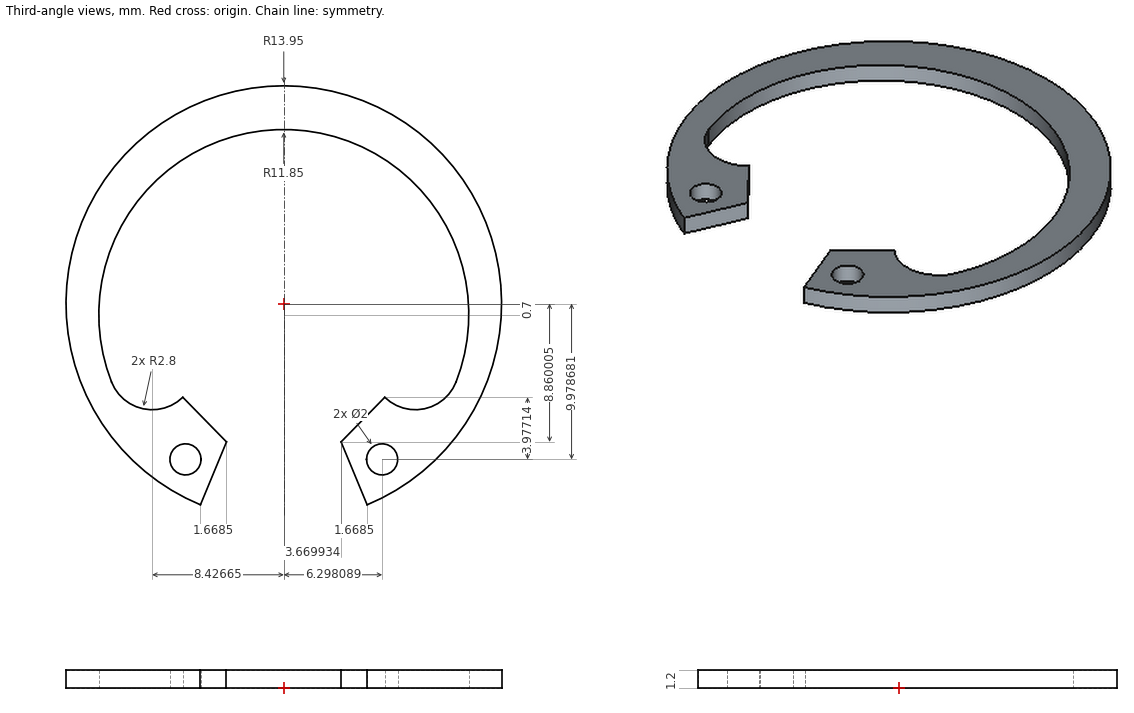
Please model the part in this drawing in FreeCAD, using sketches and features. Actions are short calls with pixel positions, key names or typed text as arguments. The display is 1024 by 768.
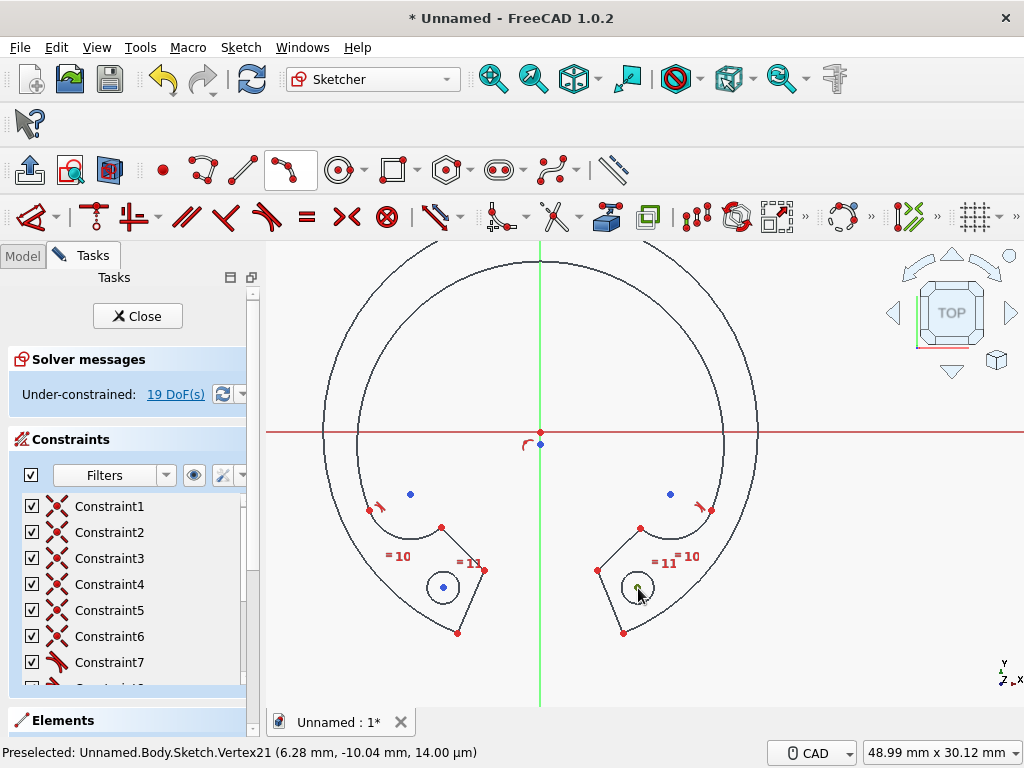
click(443, 588)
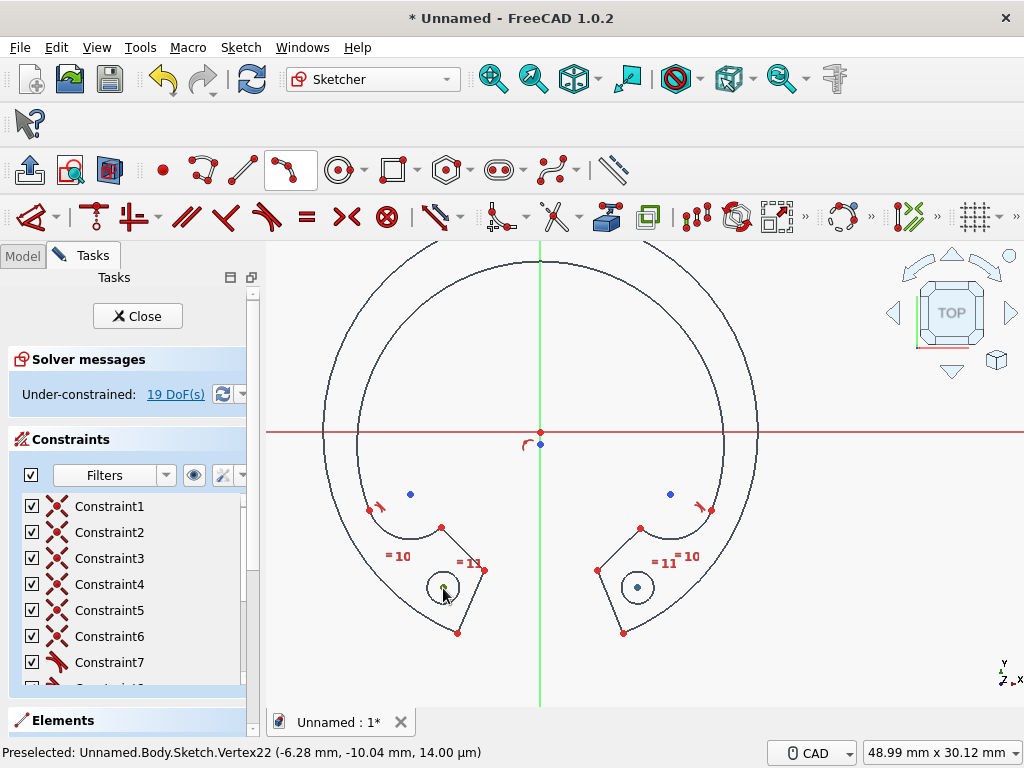
click(541, 650)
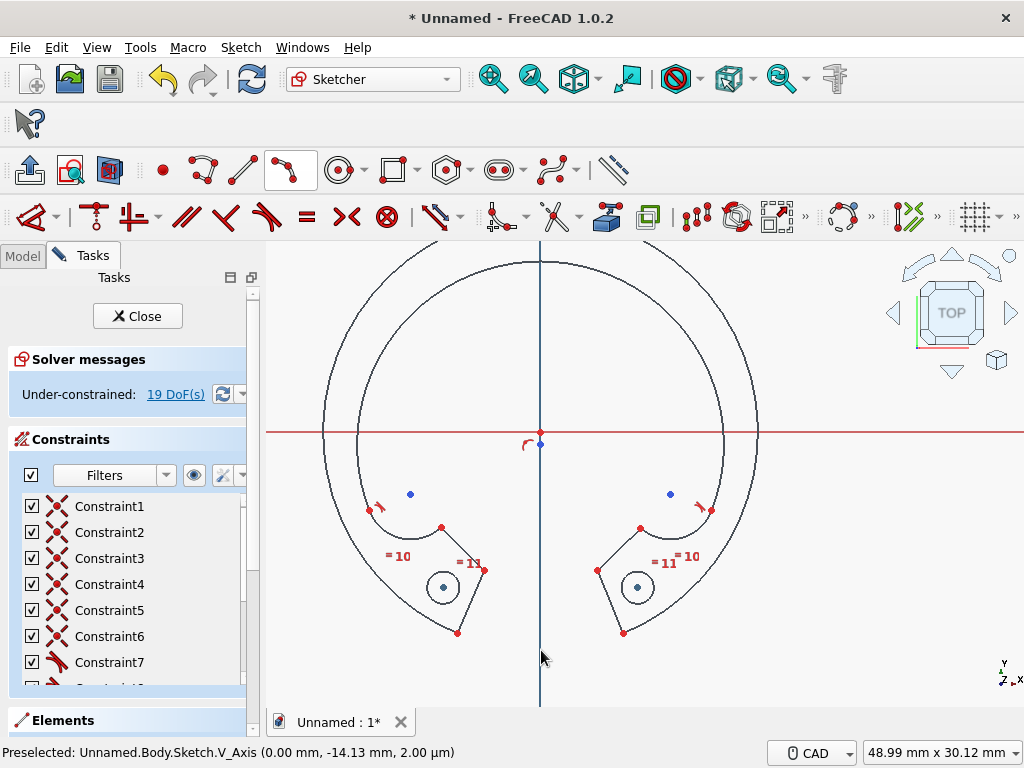
click(348, 218)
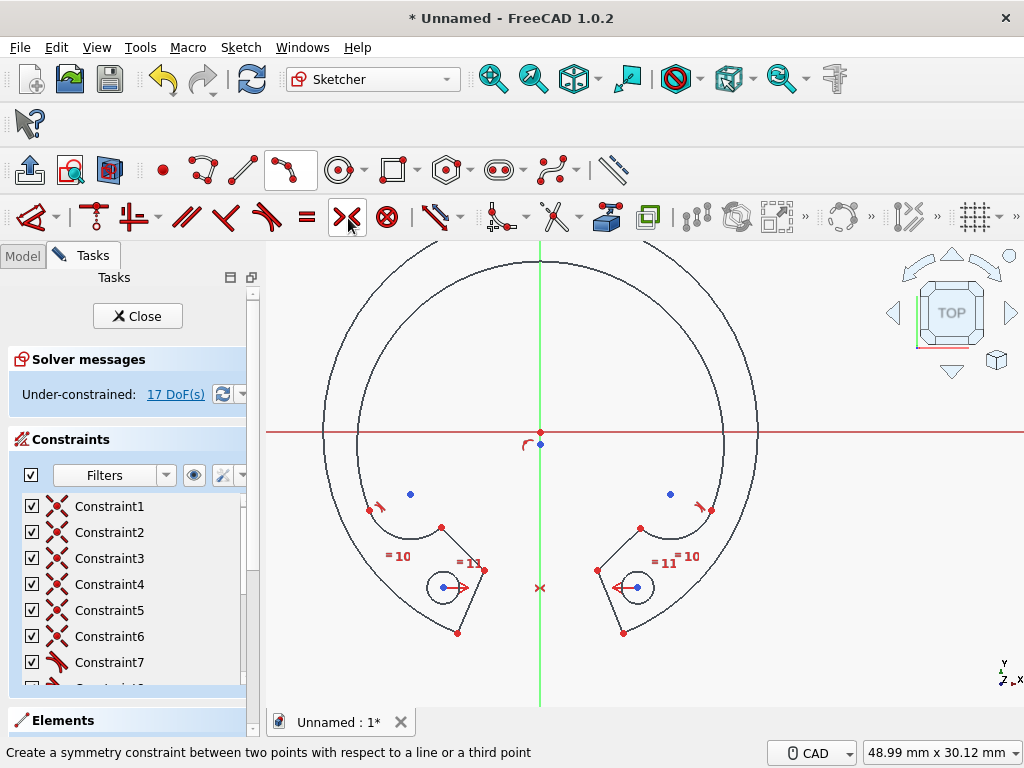
click(598, 571)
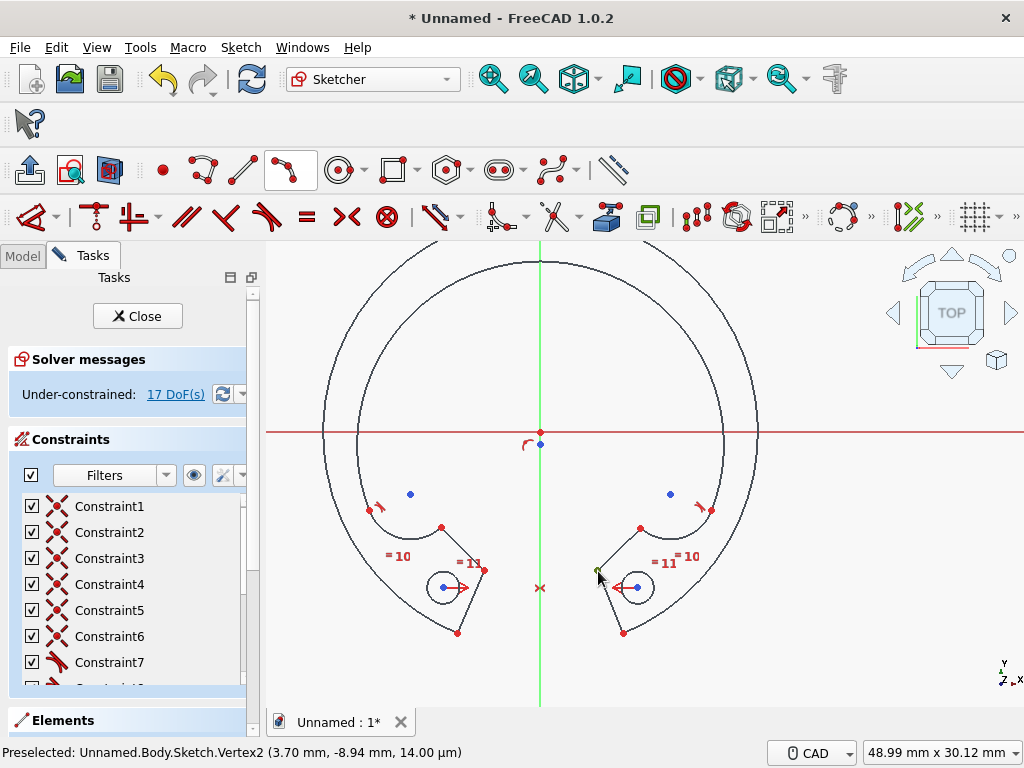
click(484, 571)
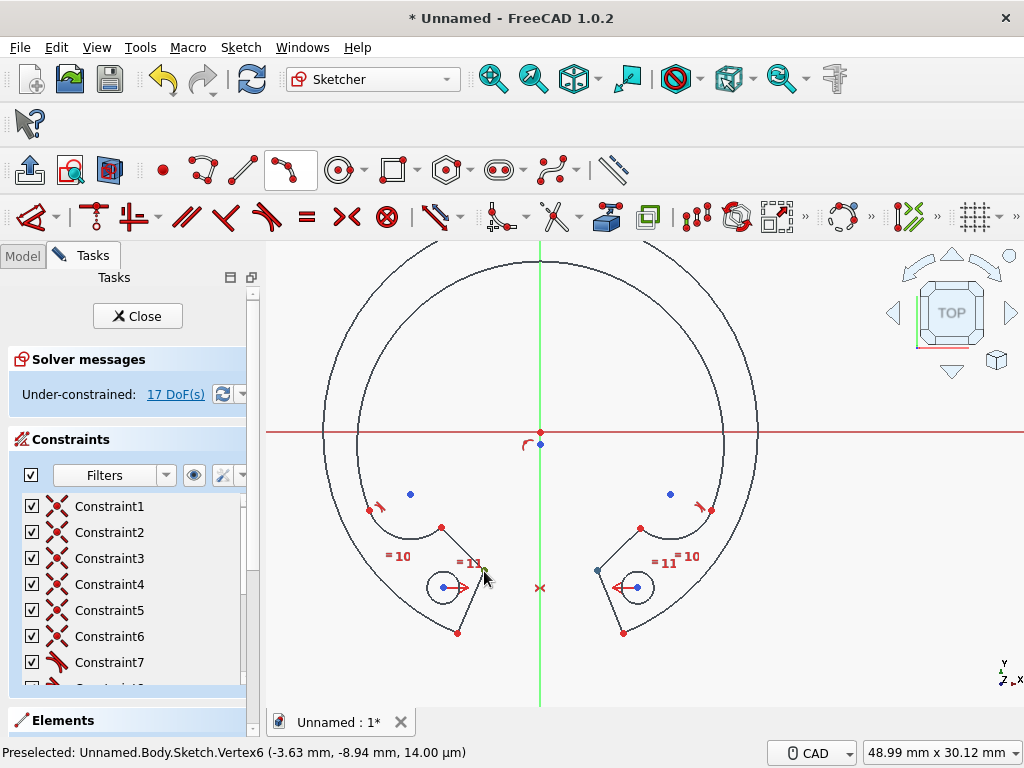
click(541, 650)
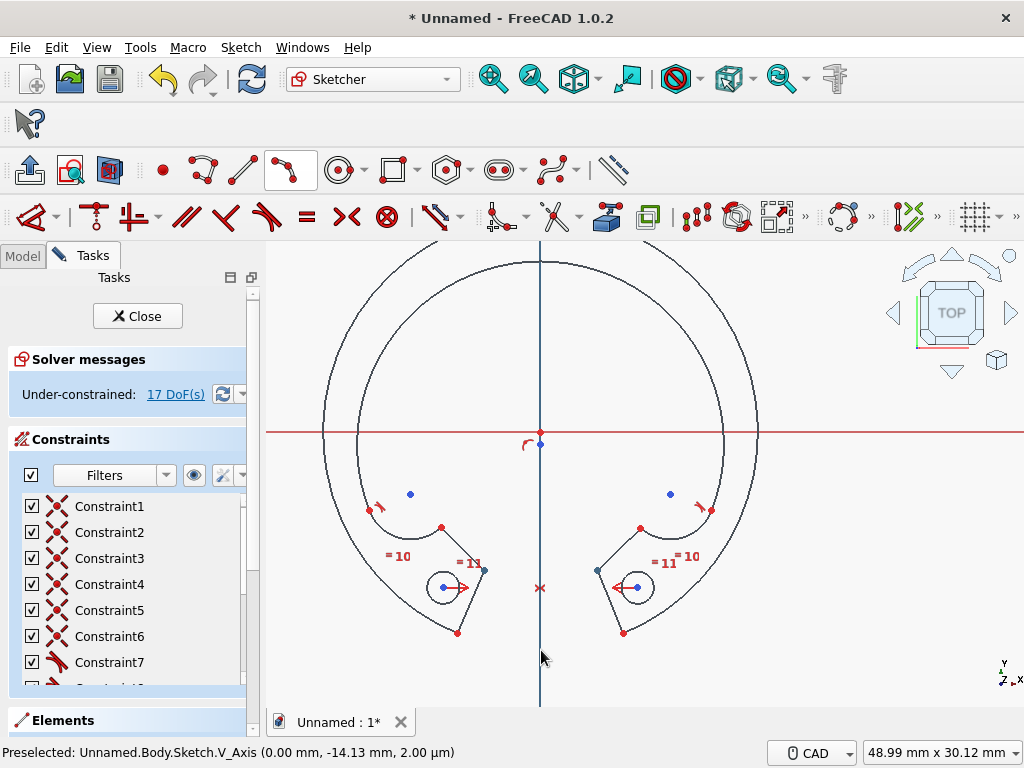
click(348, 218)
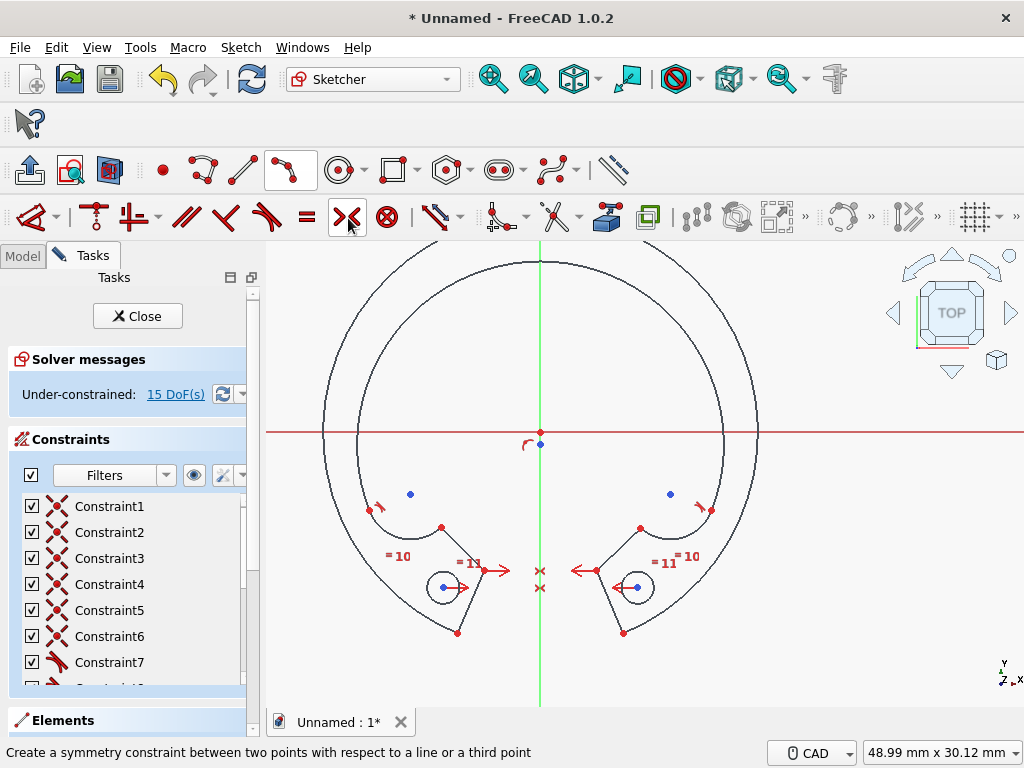
click(641, 528)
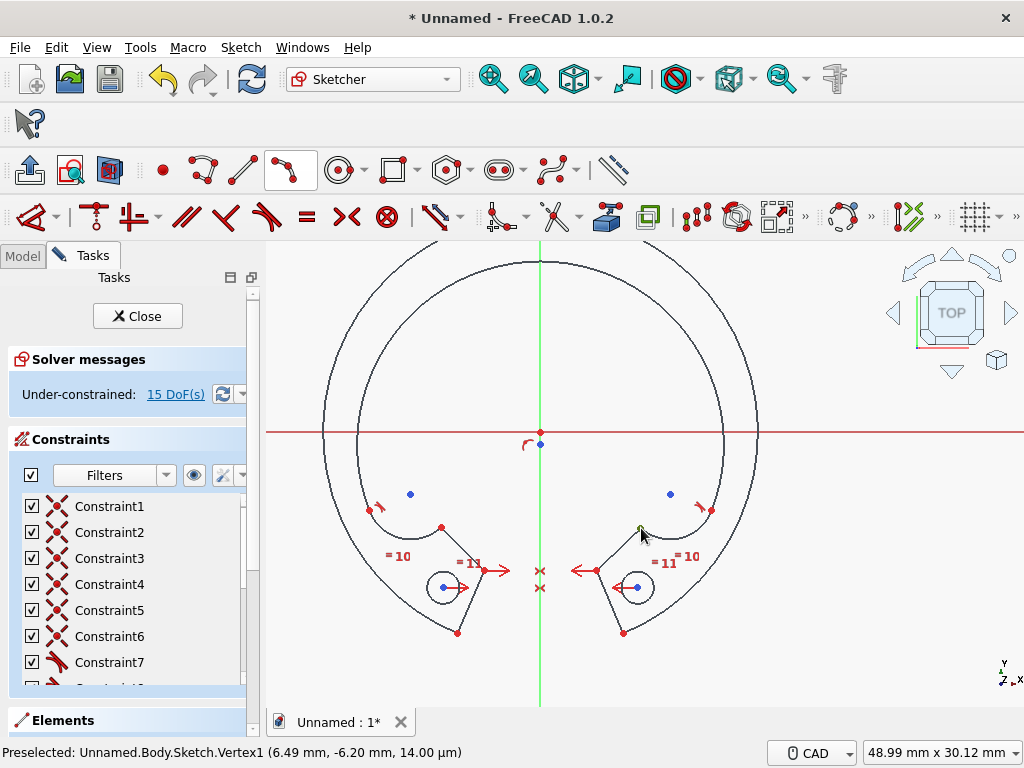
click(441, 527)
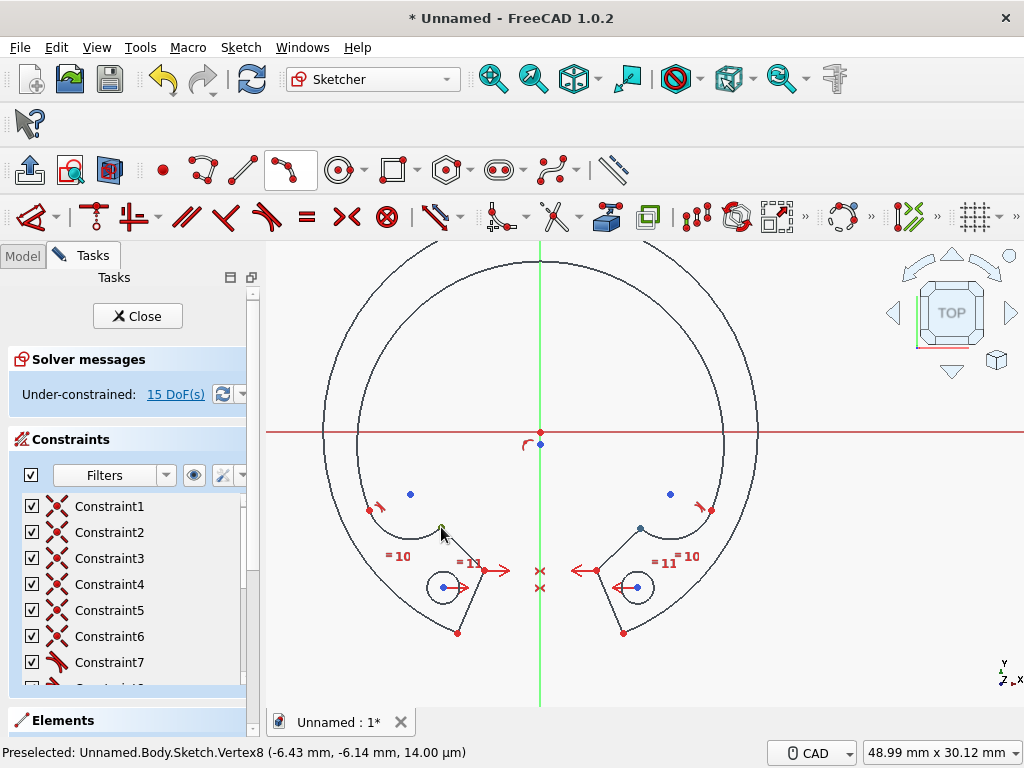
click(541, 650)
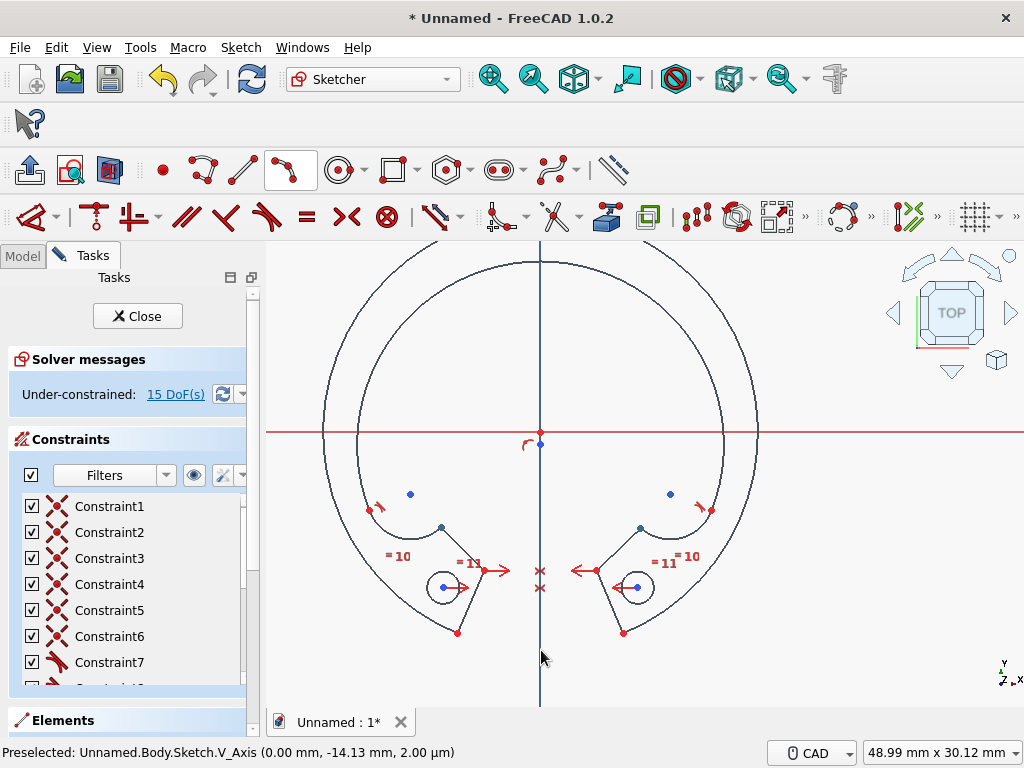
click(348, 218)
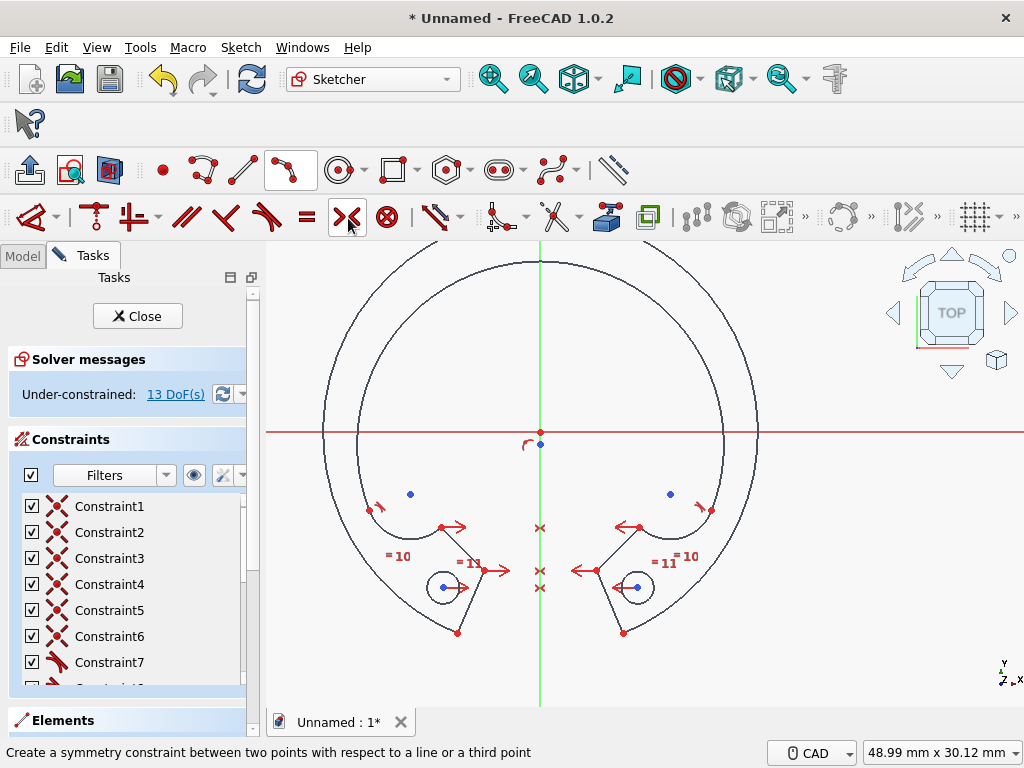
click(32, 218)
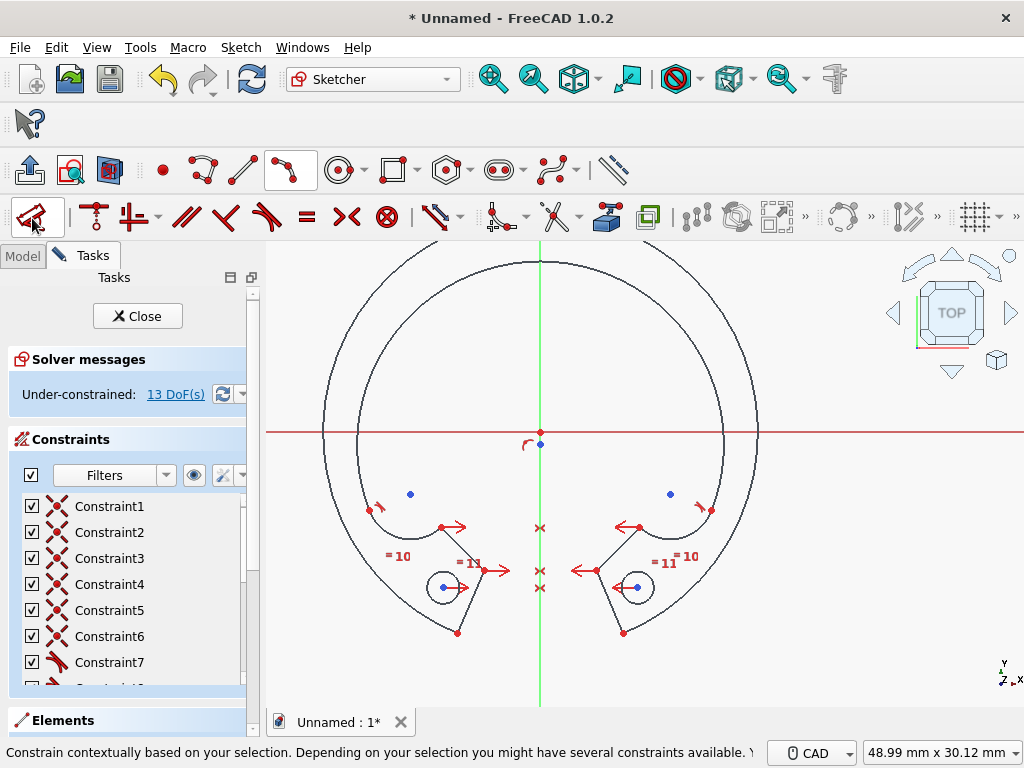
click(734, 334)
click(763, 319)